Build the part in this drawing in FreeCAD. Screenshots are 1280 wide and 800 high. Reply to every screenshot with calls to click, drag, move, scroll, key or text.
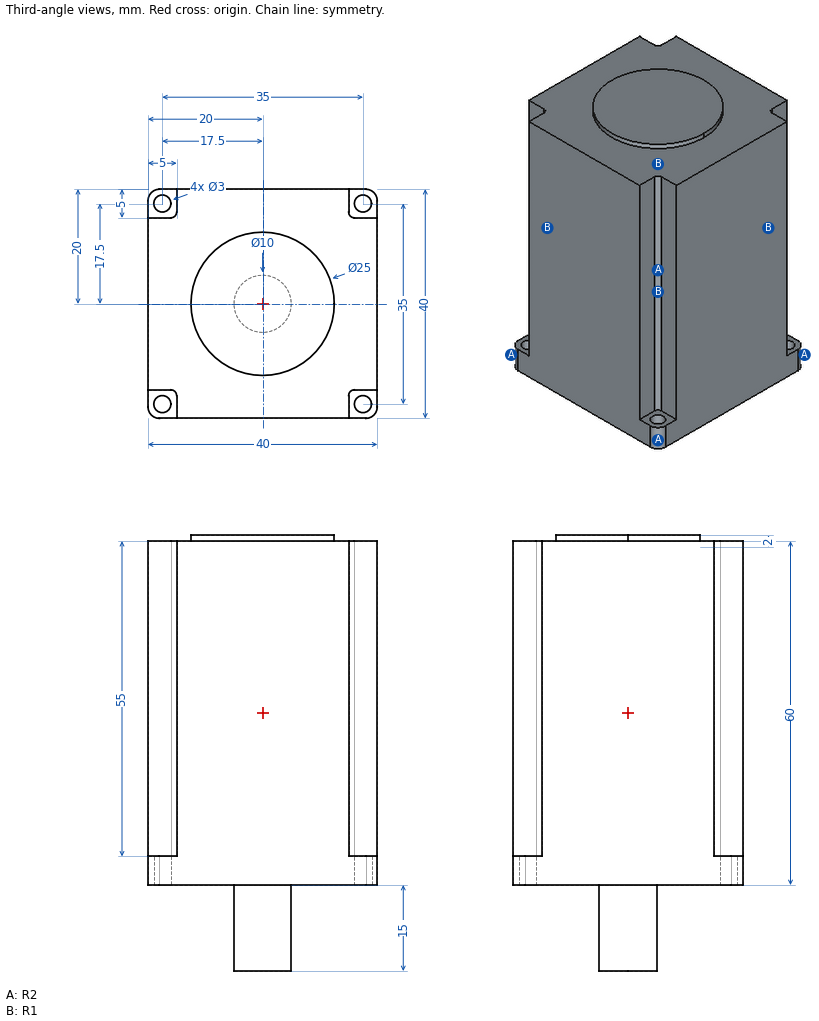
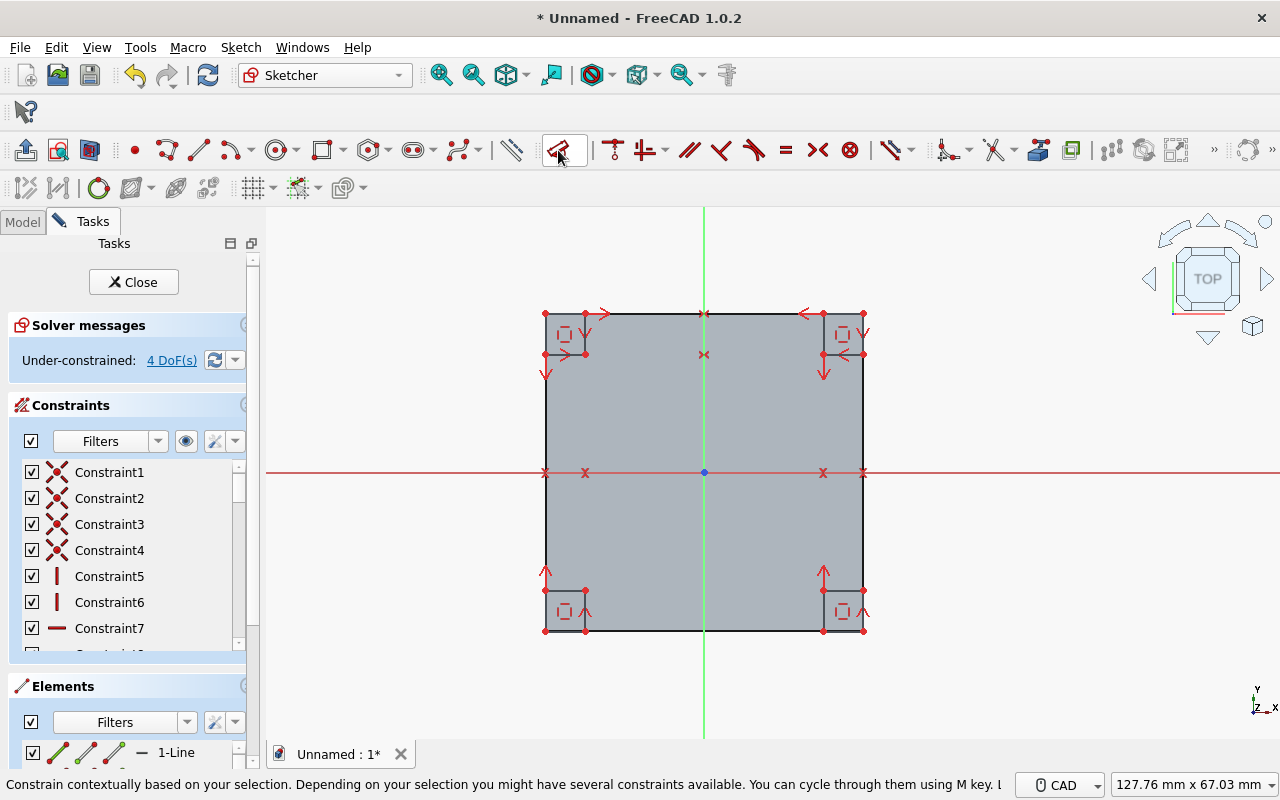
click(546, 326)
click(512, 334)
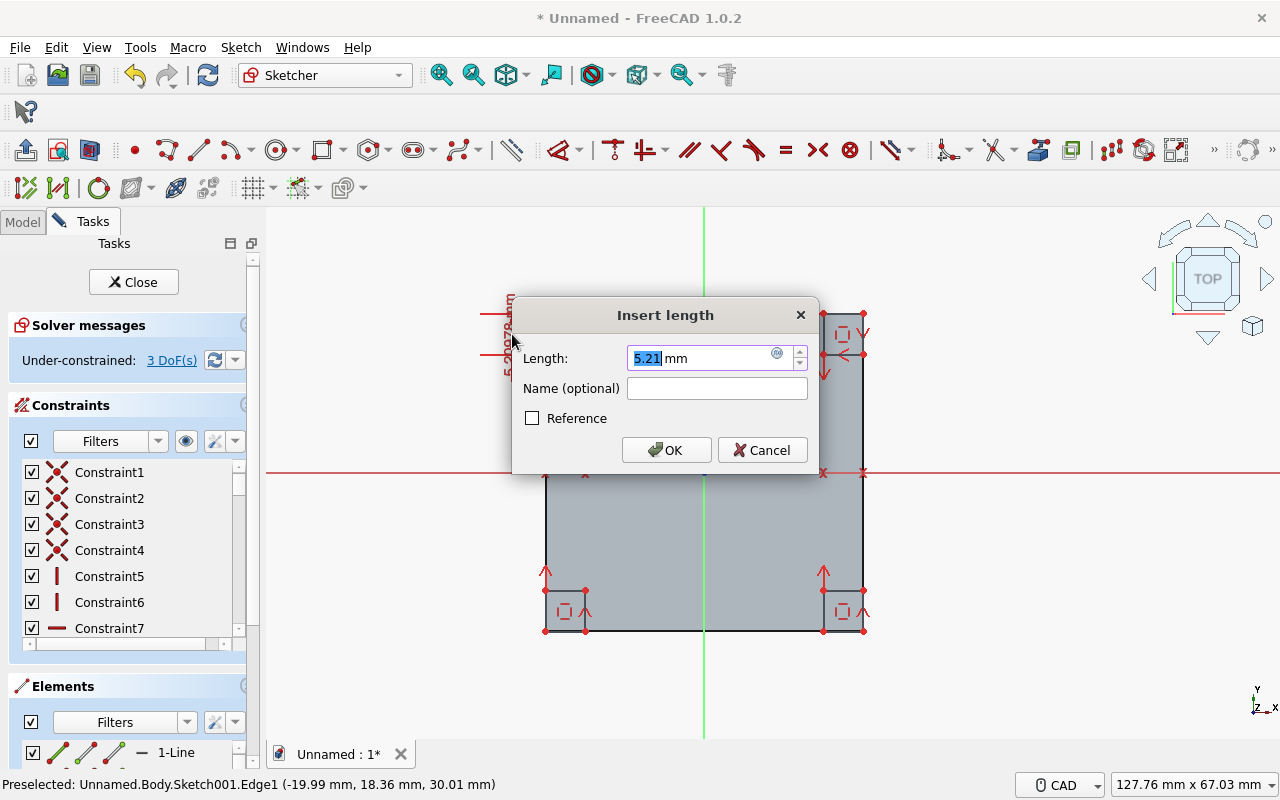
text(5)
key(Return)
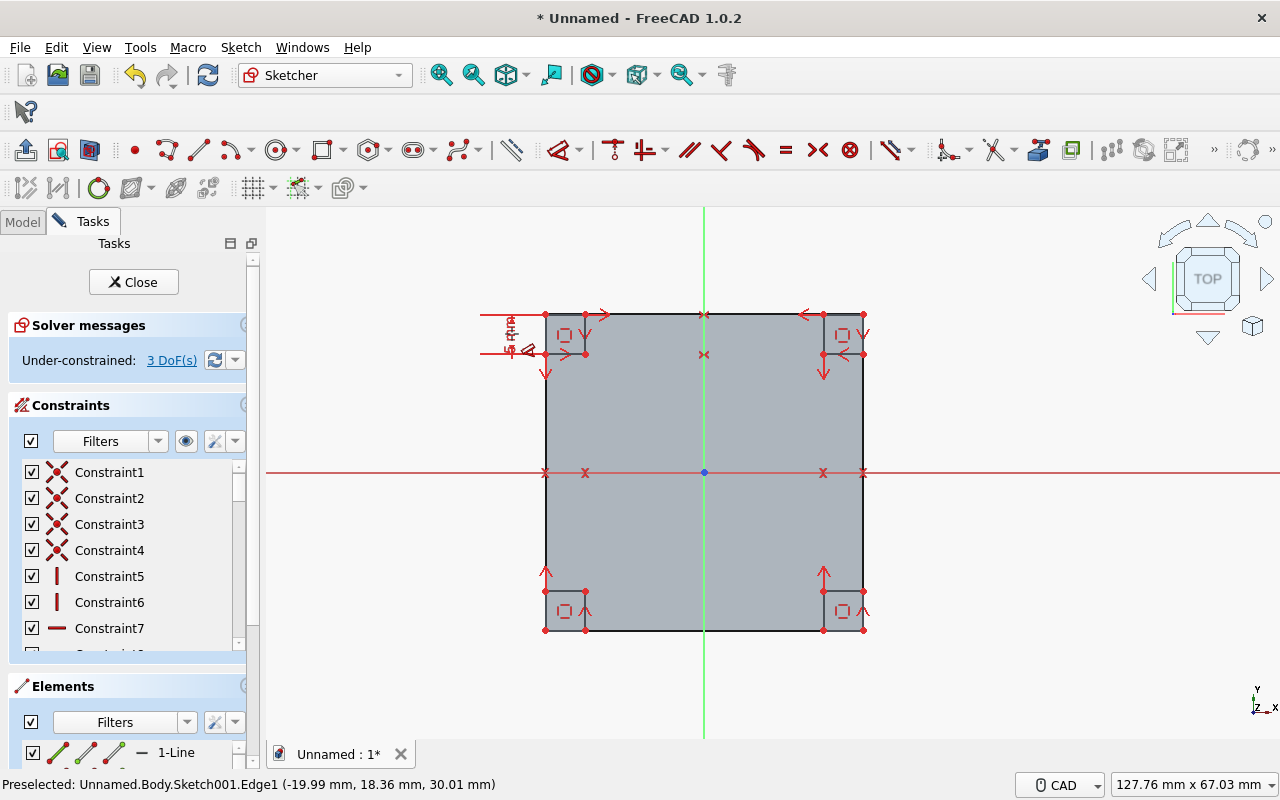
click(557, 354)
click(565, 388)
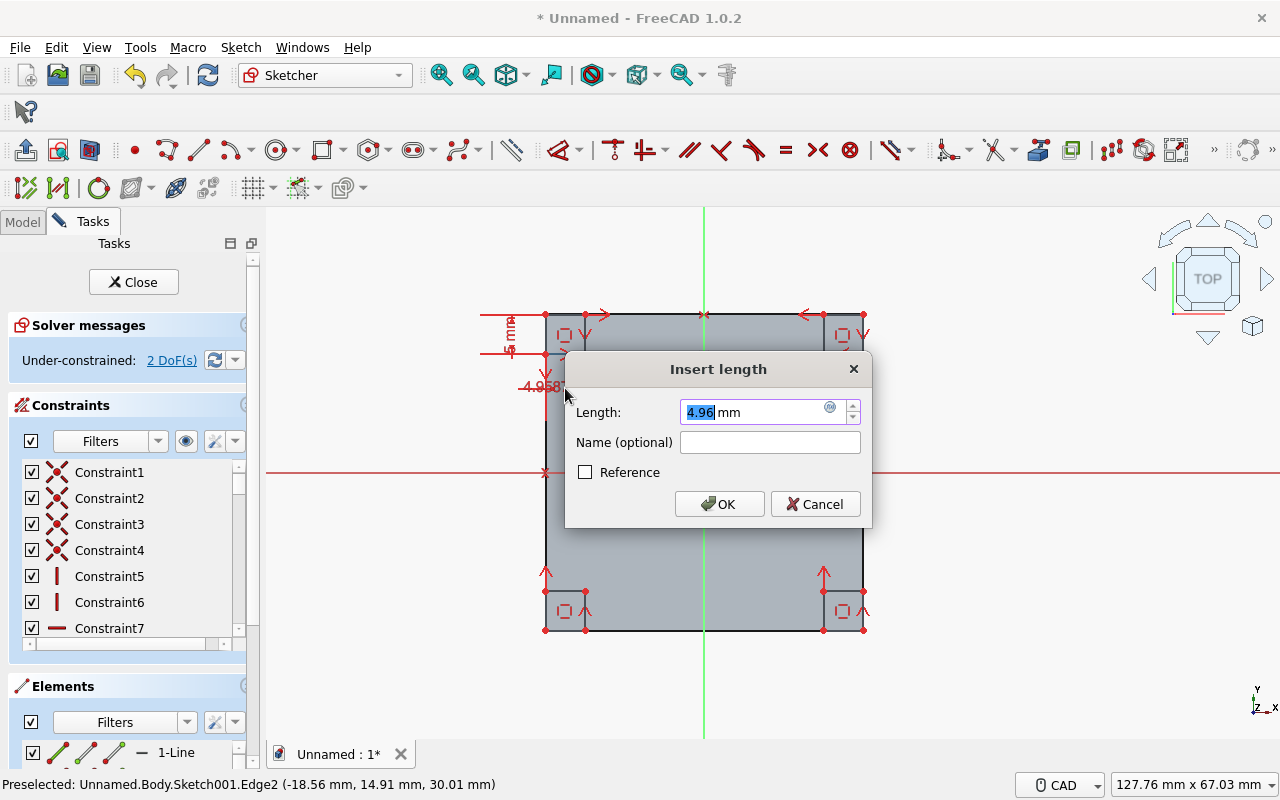
text(5)
key(Return)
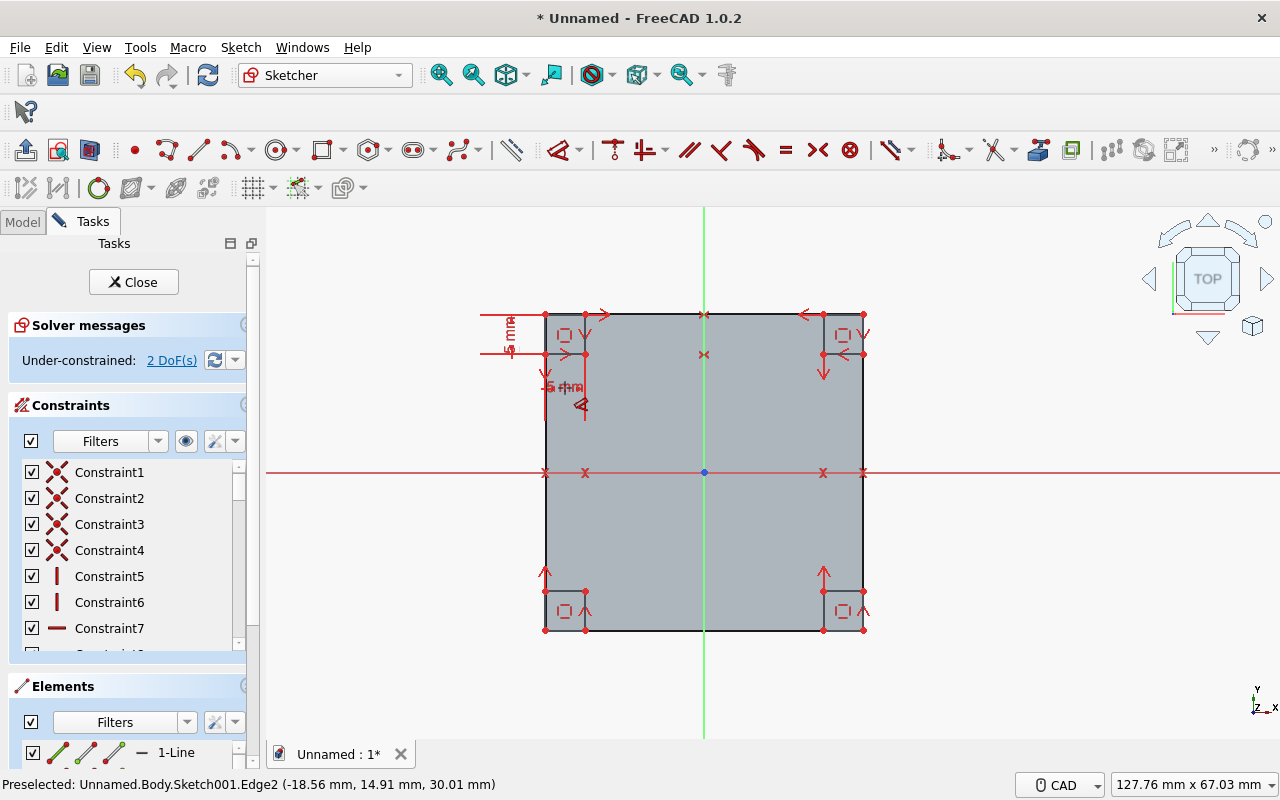
click(545, 315)
click(625, 281)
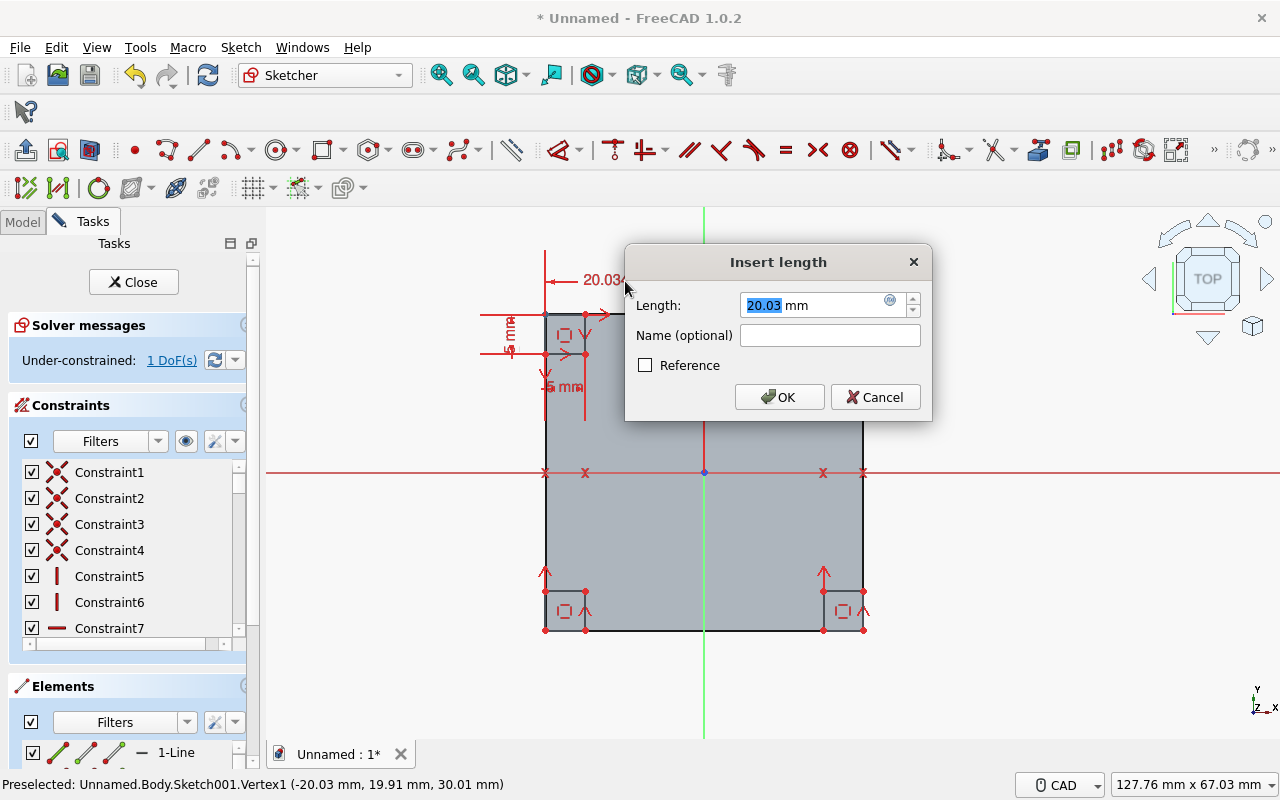
text(20)
key(Return)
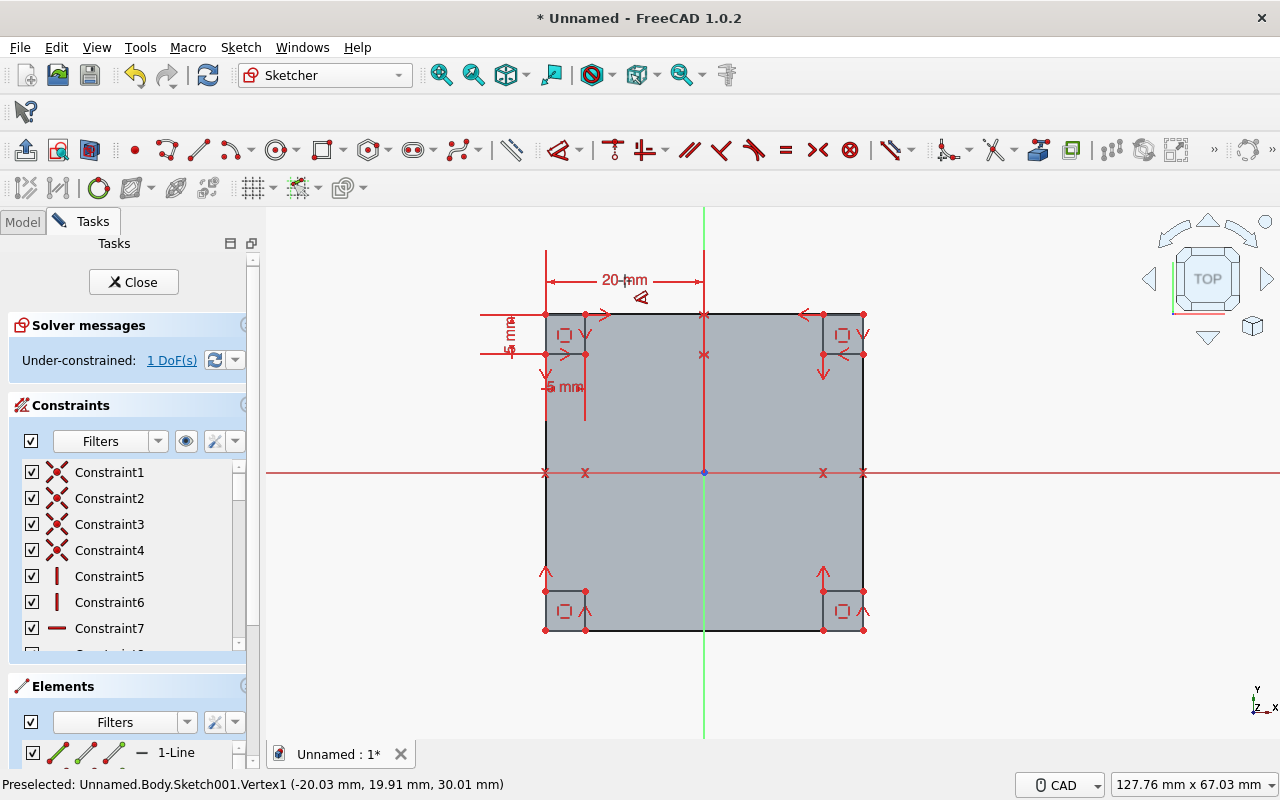
click(546, 315)
click(512, 357)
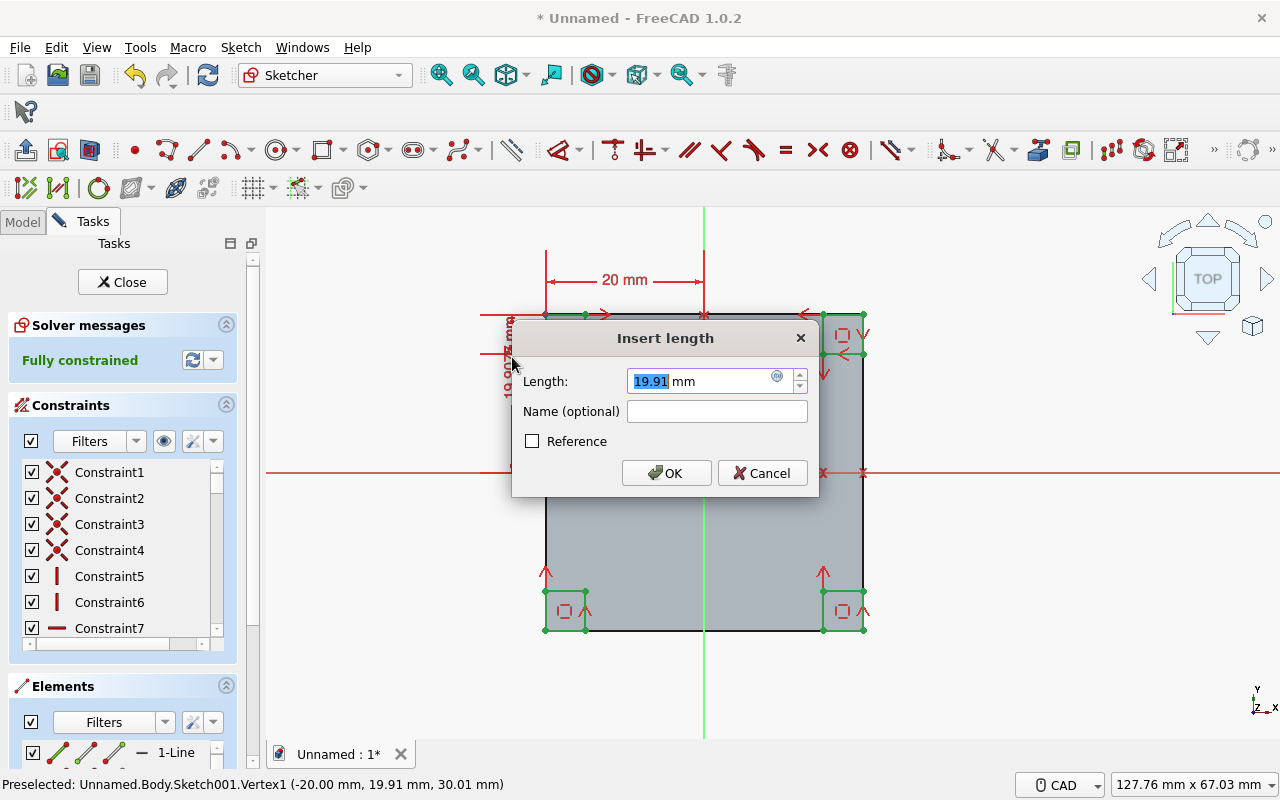
text(20)
key(Return)
key(Escape)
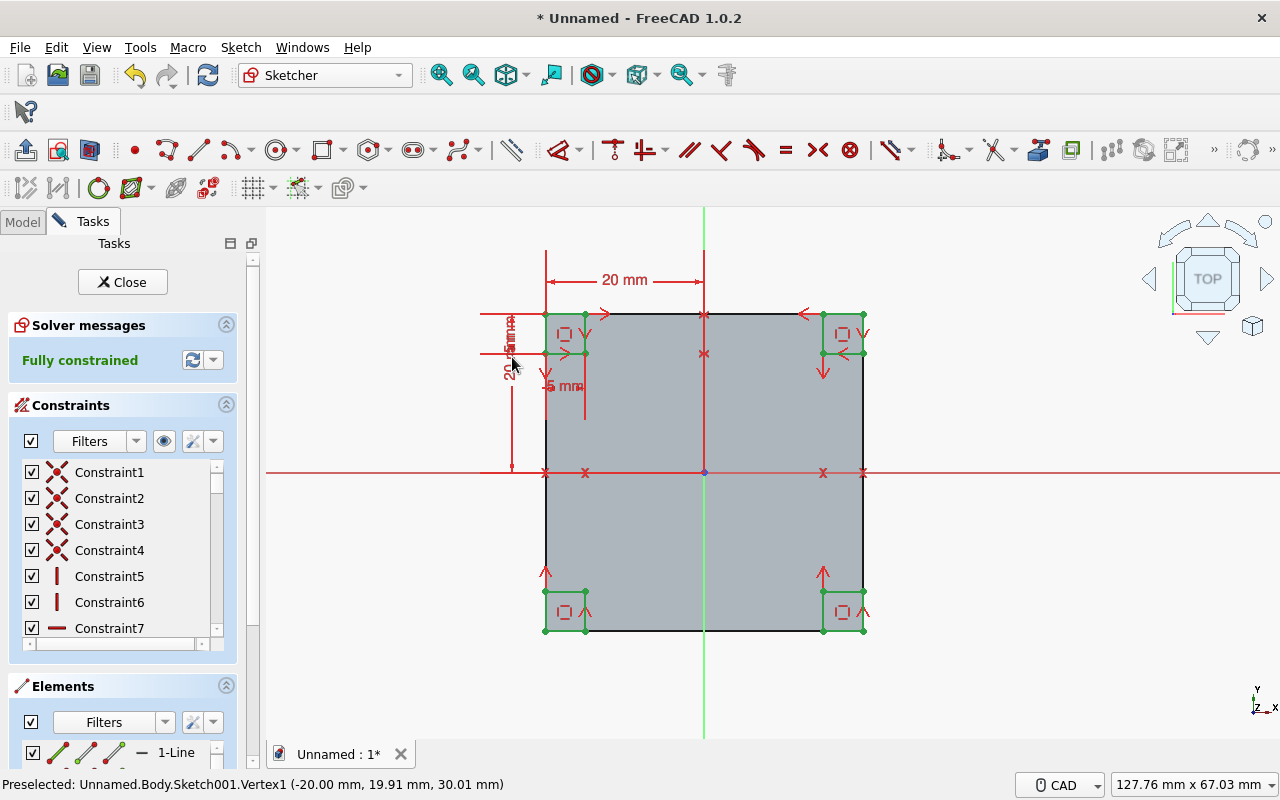
click(123, 282)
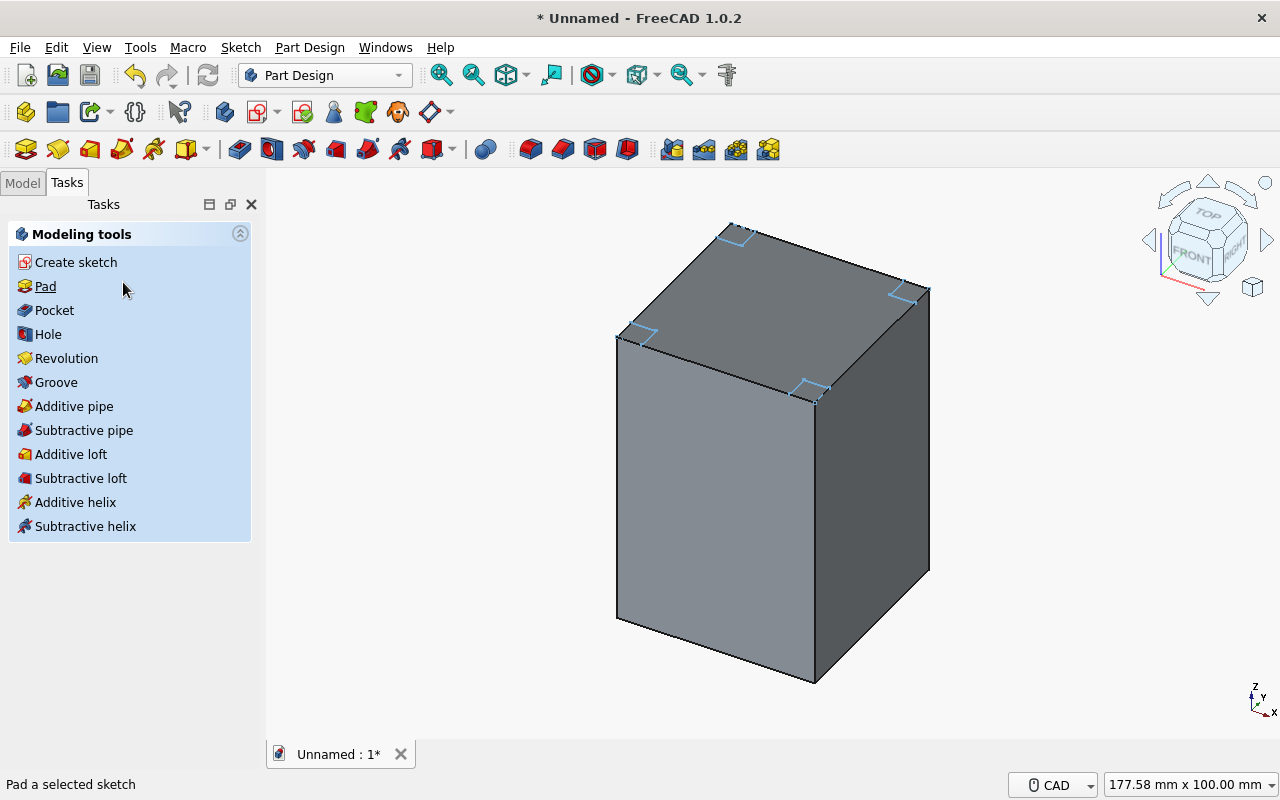
click(240, 150)